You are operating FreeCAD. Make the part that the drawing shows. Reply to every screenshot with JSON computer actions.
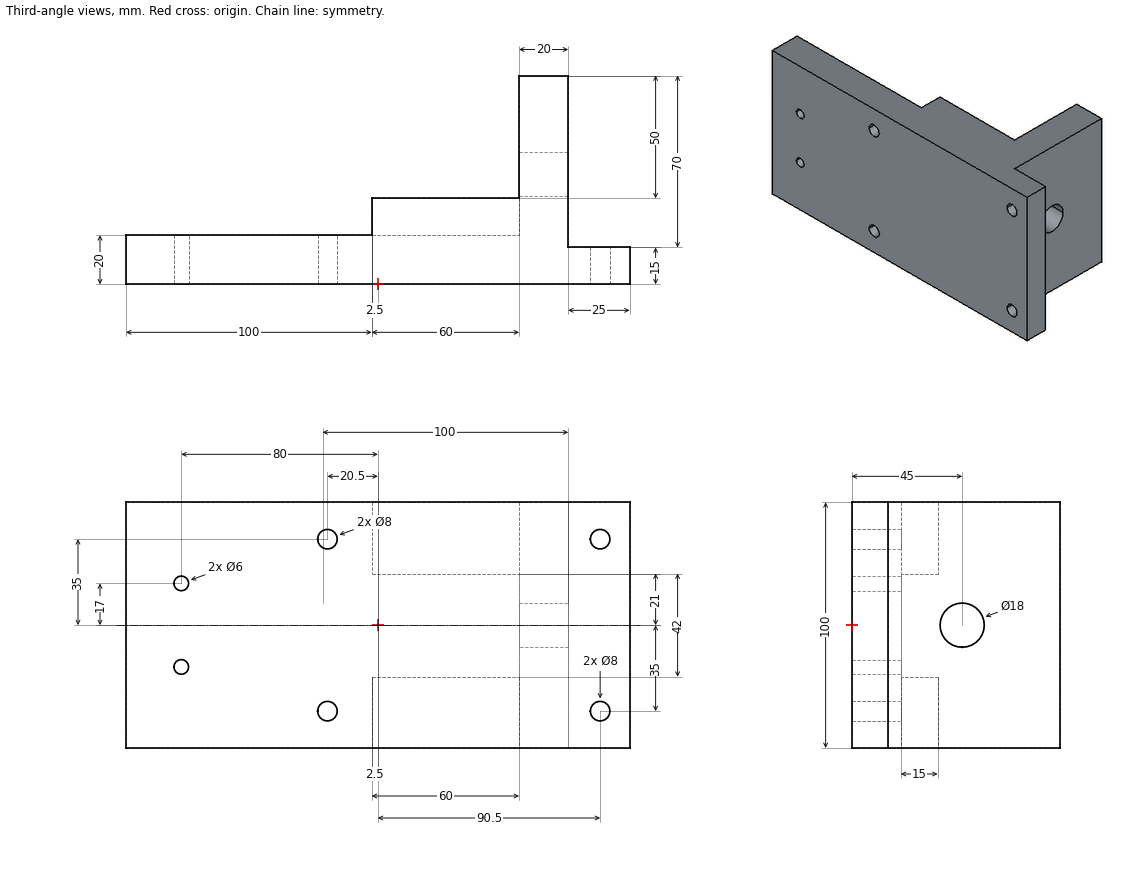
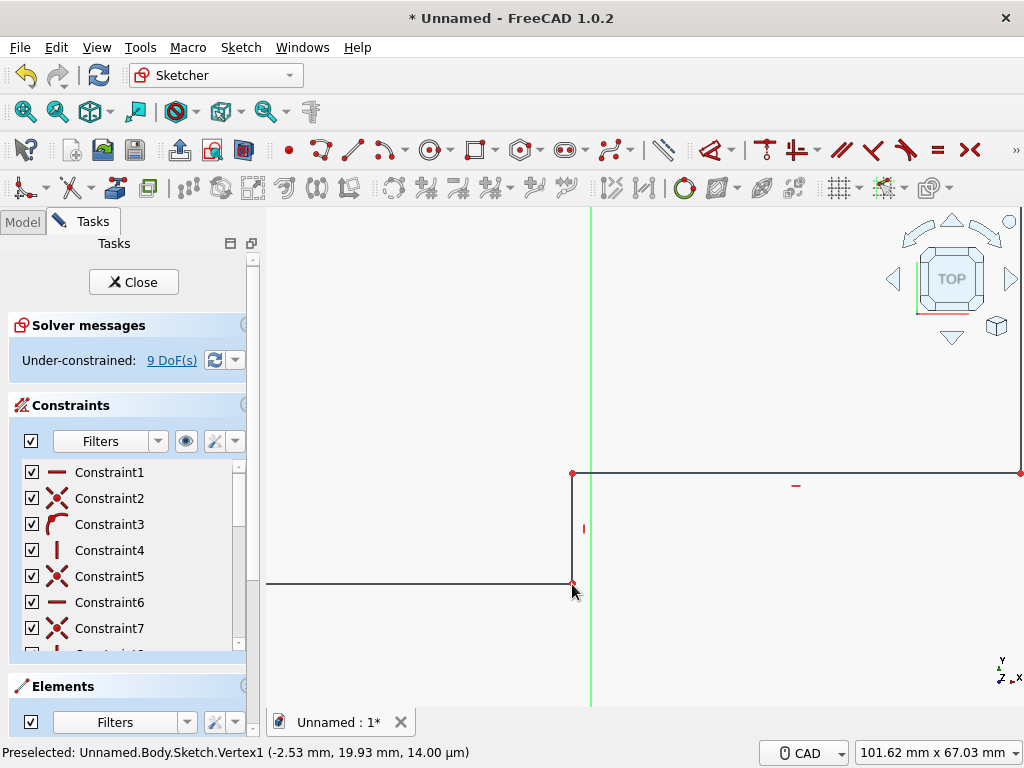
{"action": "left_click", "coordinate": [710, 150]}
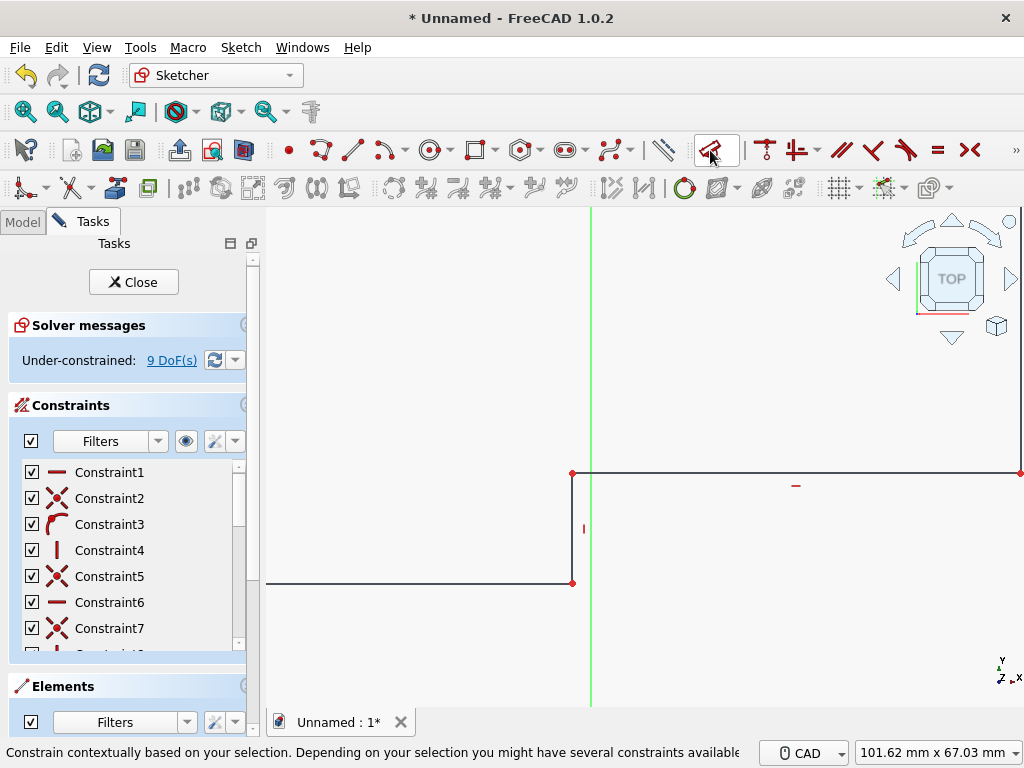
{"action": "scroll", "coordinate": [572, 471], "scroll_direction": "down", "scroll_amount": 7}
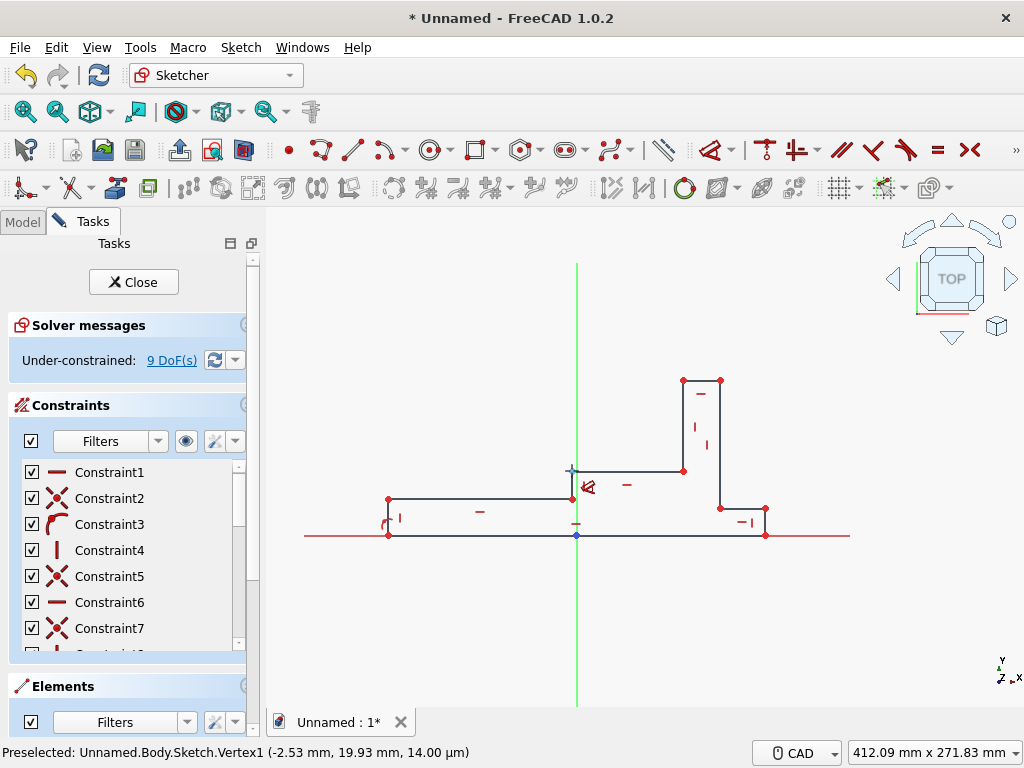
{"action": "scroll", "coordinate": [388, 510], "scroll_direction": "up", "scroll_amount": 2}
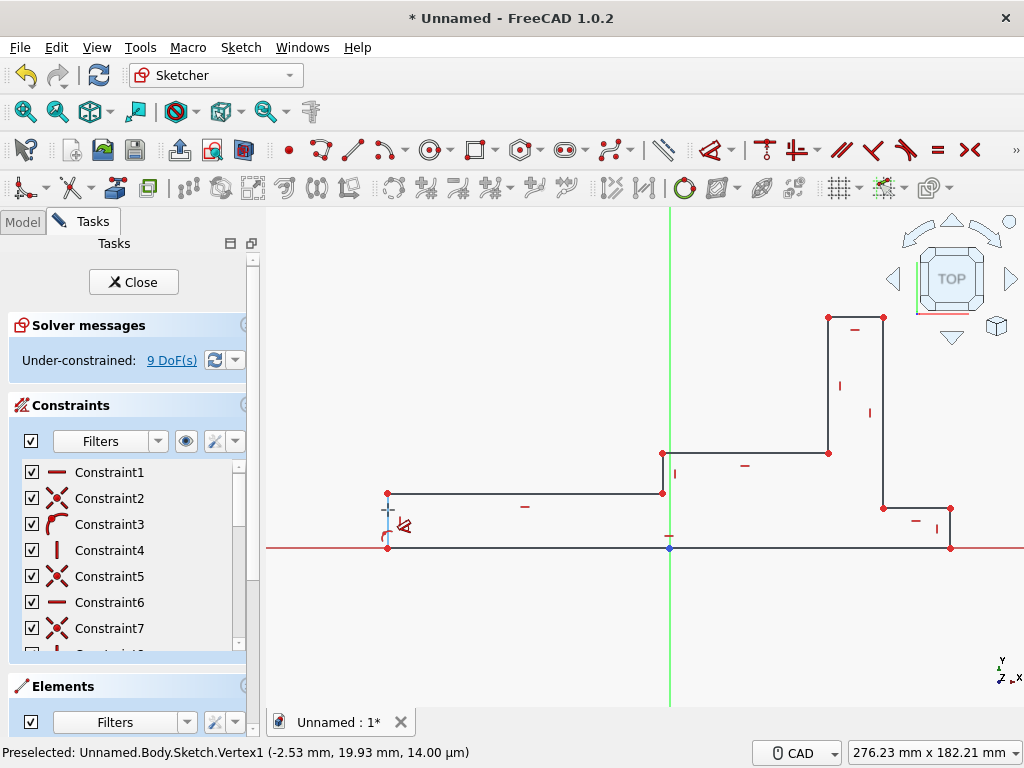
{"action": "left_click", "coordinate": [388, 510]}
{"action": "left_click", "coordinate": [354, 521]}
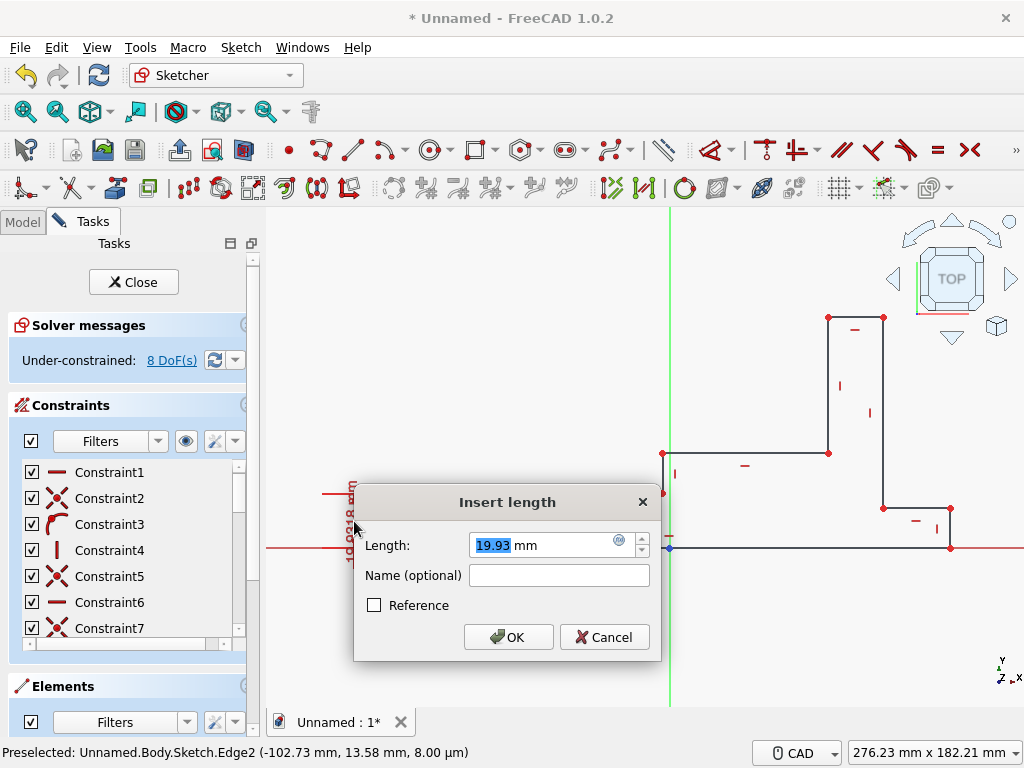
{"action": "type", "text": "20"}
{"action": "key", "text": "Return"}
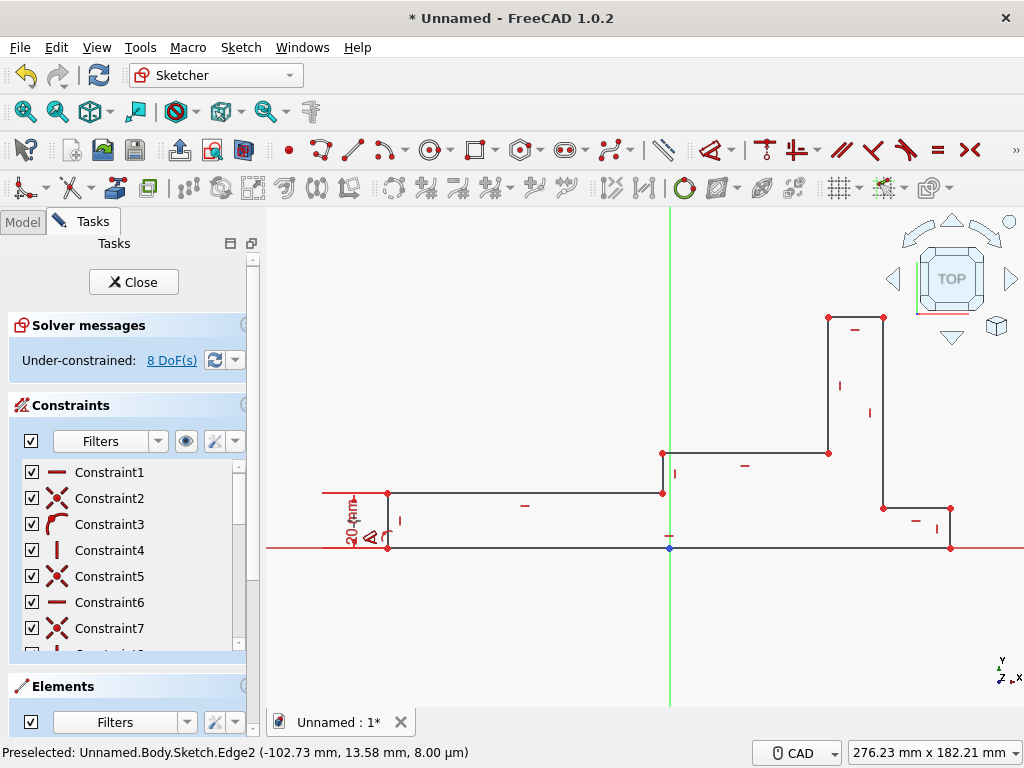
{"action": "scroll", "coordinate": [387, 509], "scroll_direction": "down", "scroll_amount": 2}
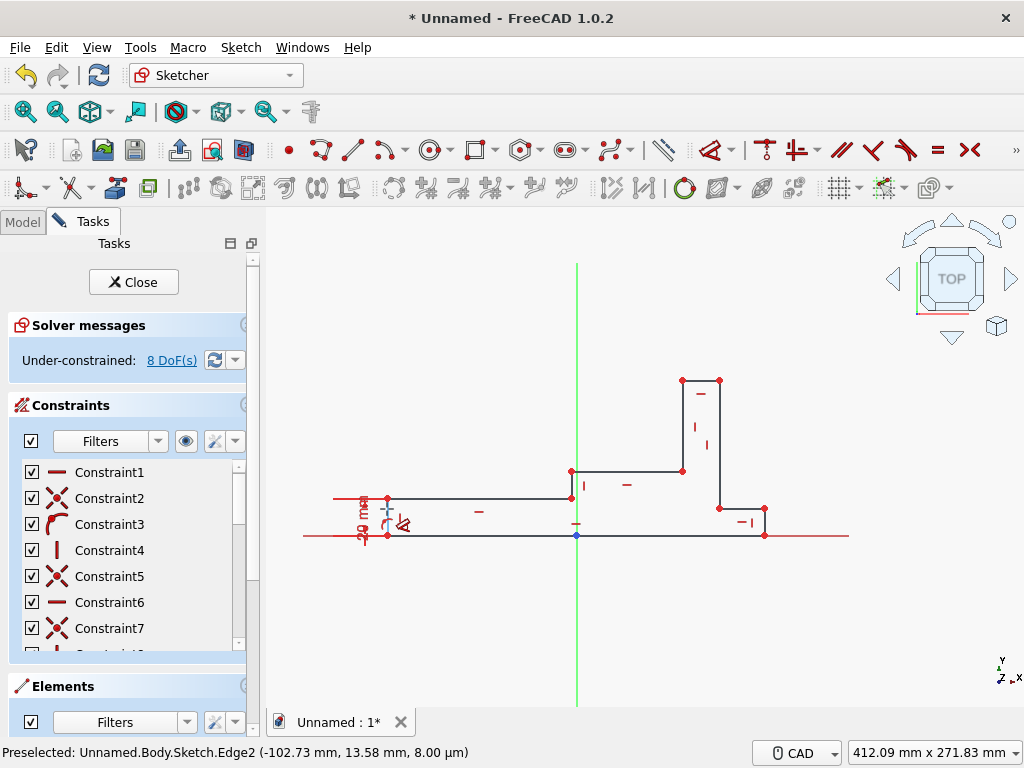
{"action": "scroll", "coordinate": [765, 527], "scroll_direction": "up", "scroll_amount": 3}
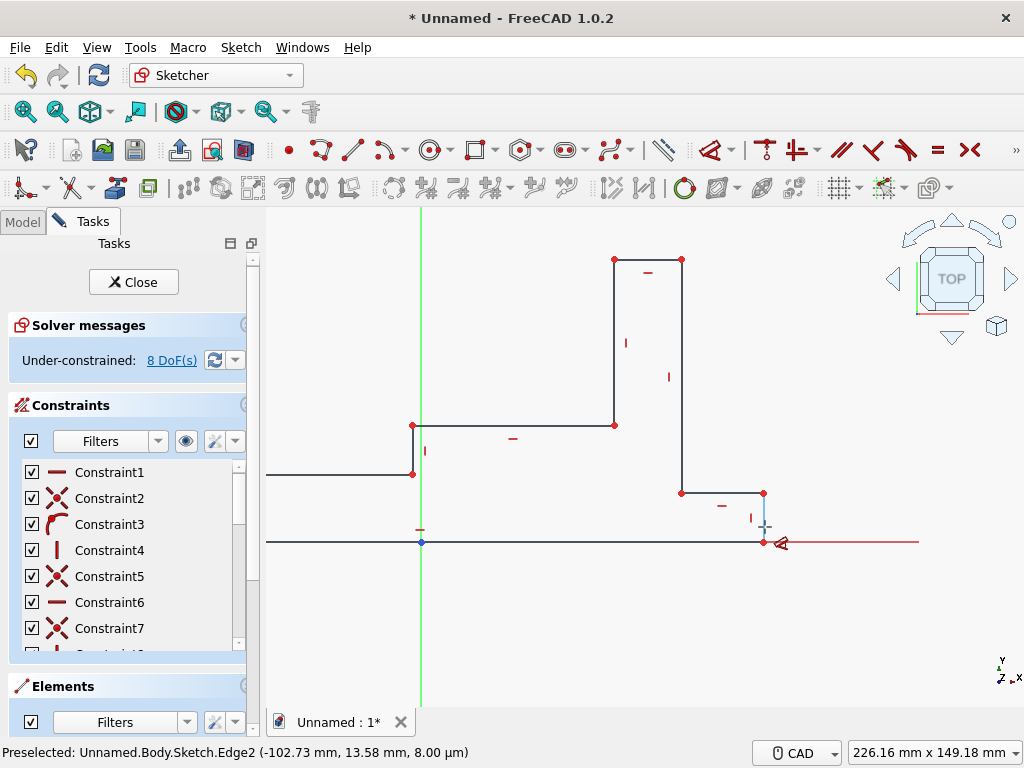
{"action": "left_click", "coordinate": [764, 527]}
{"action": "left_click", "coordinate": [798, 518]}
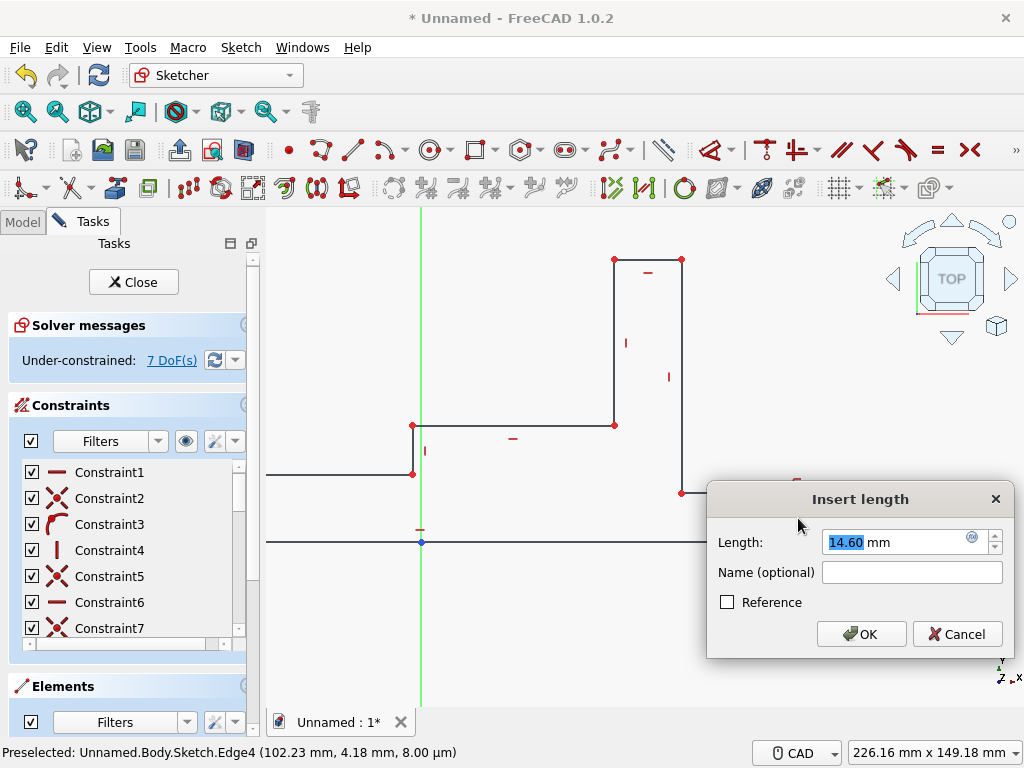
{"action": "type", "text": "15"}
{"action": "key", "text": "Return"}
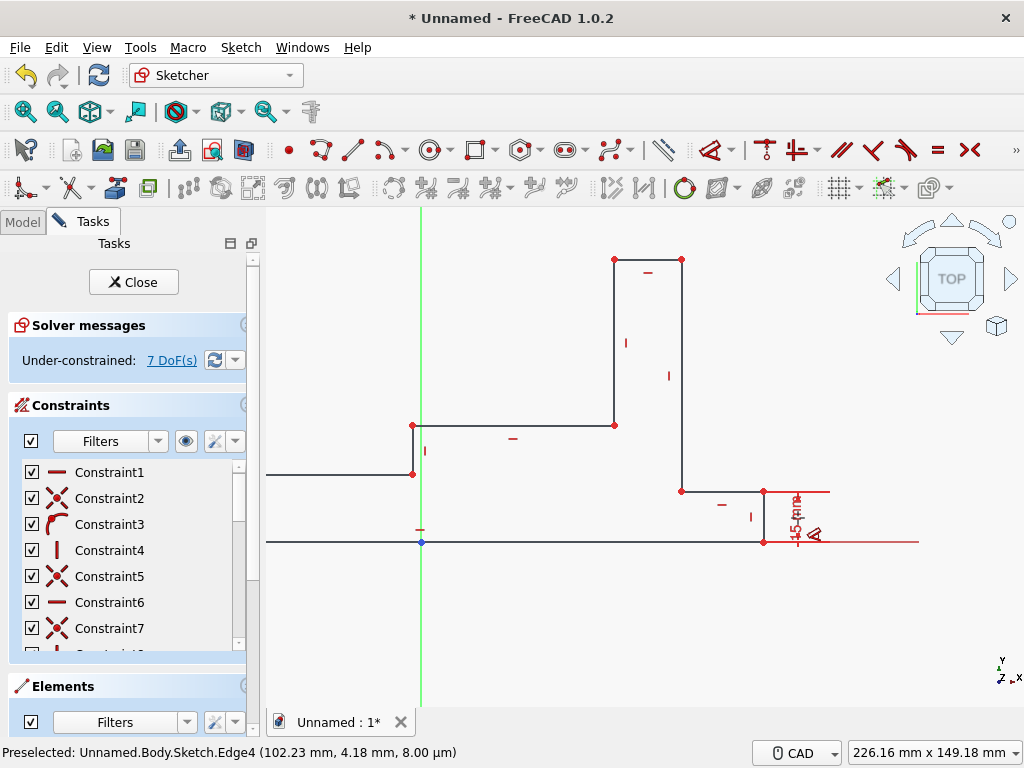
{"action": "left_click", "coordinate": [739, 492]}
{"action": "left_click", "coordinate": [723, 526]}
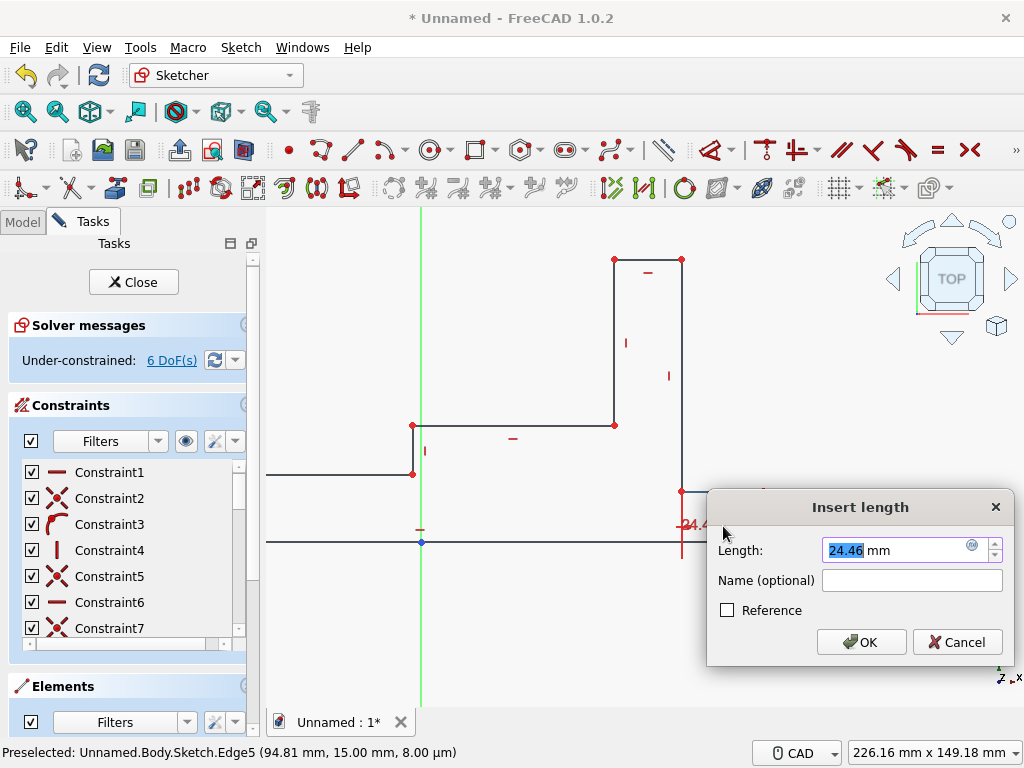
{"action": "type", "text": "25"}
{"action": "key", "text": "Return"}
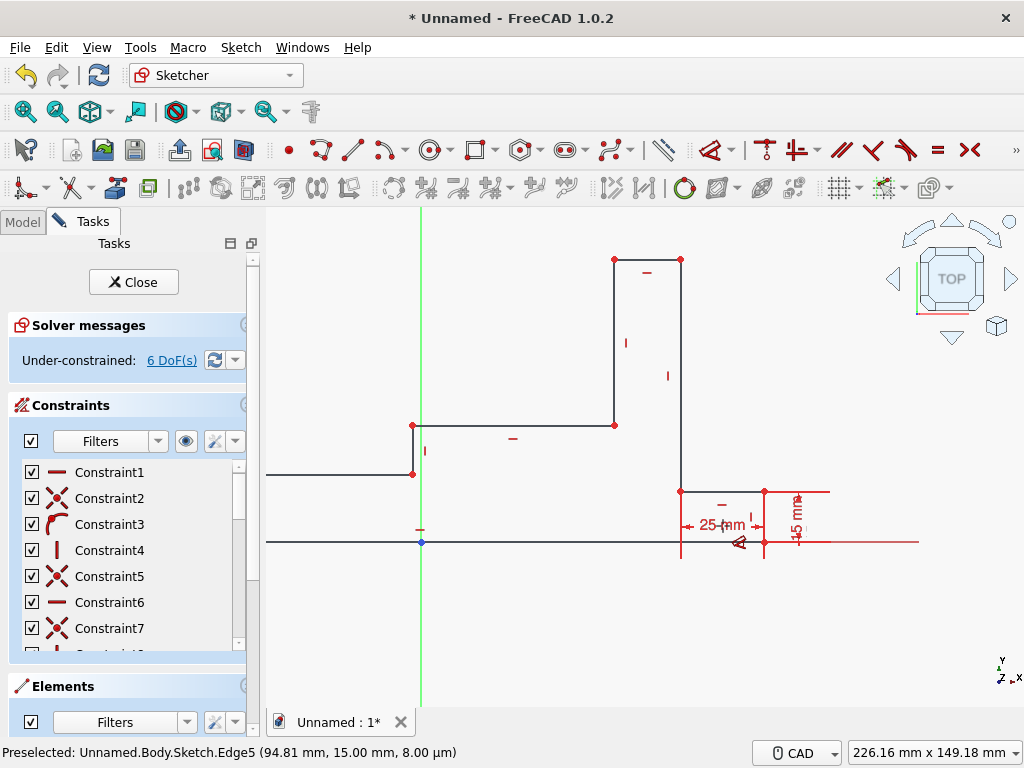
{"action": "left_click", "coordinate": [681, 422]}
{"action": "left_click", "coordinate": [715, 376]}